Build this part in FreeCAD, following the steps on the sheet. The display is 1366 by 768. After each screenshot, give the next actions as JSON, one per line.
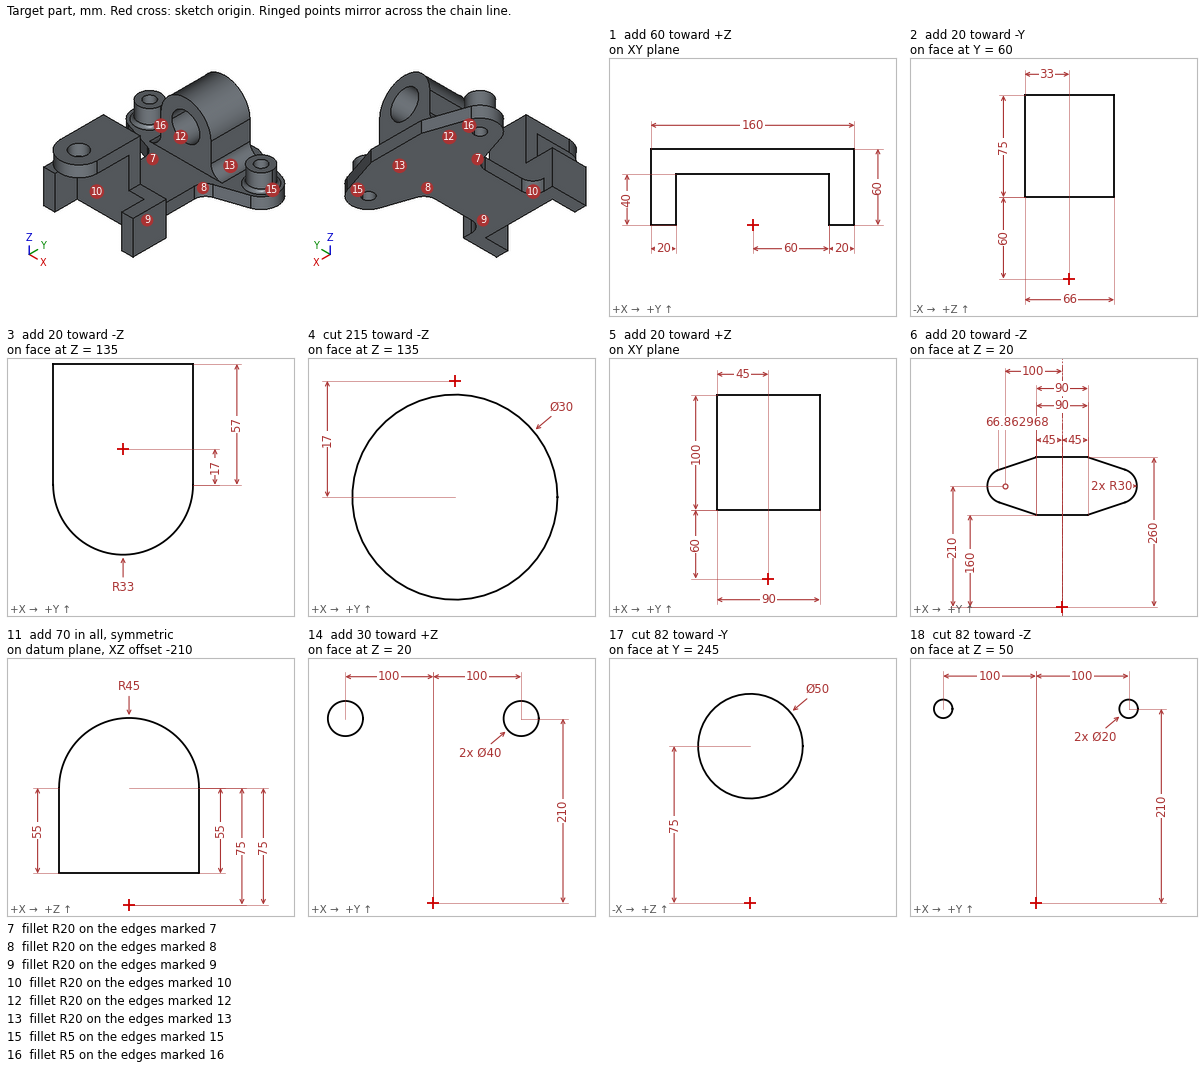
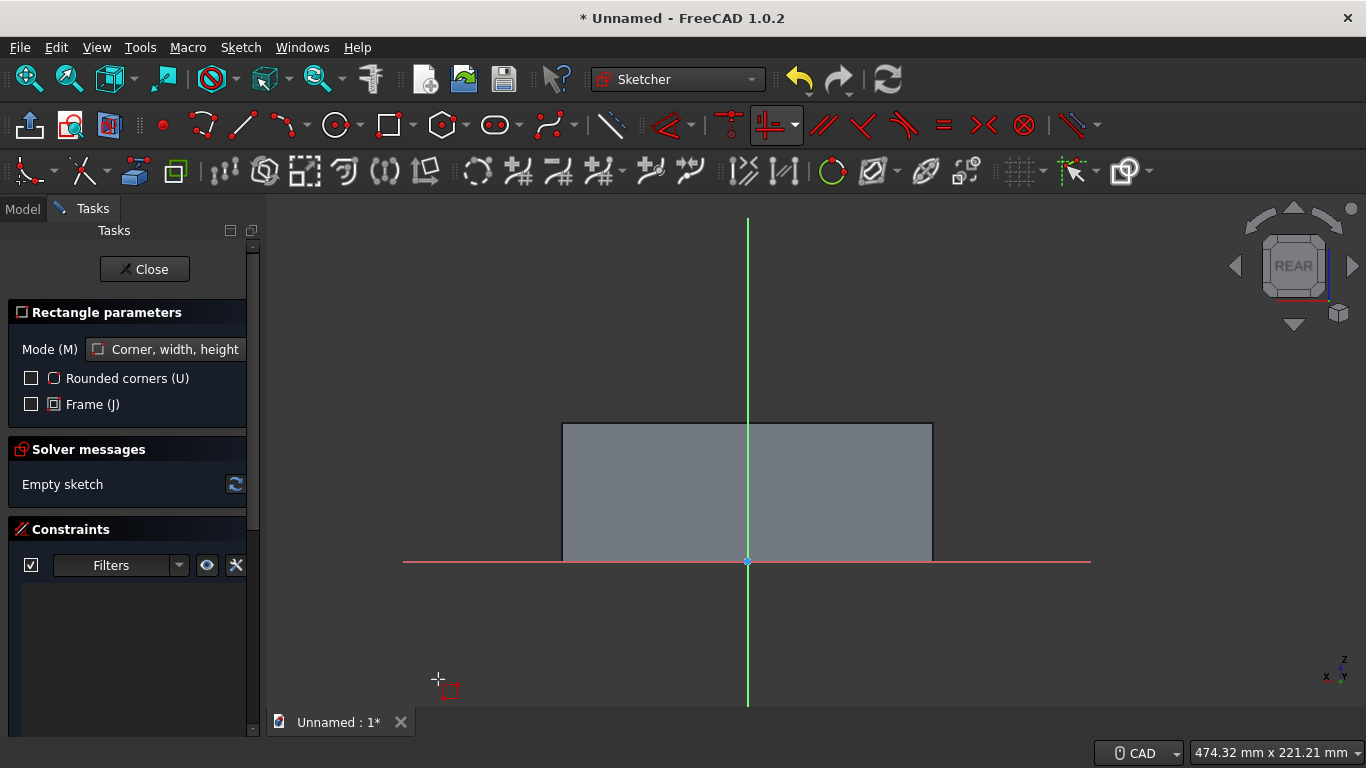
{"action": "left_click", "coordinate": [671, 249]}
{"action": "left_click", "coordinate": [824, 423]}
{"action": "key", "text": "Escape"}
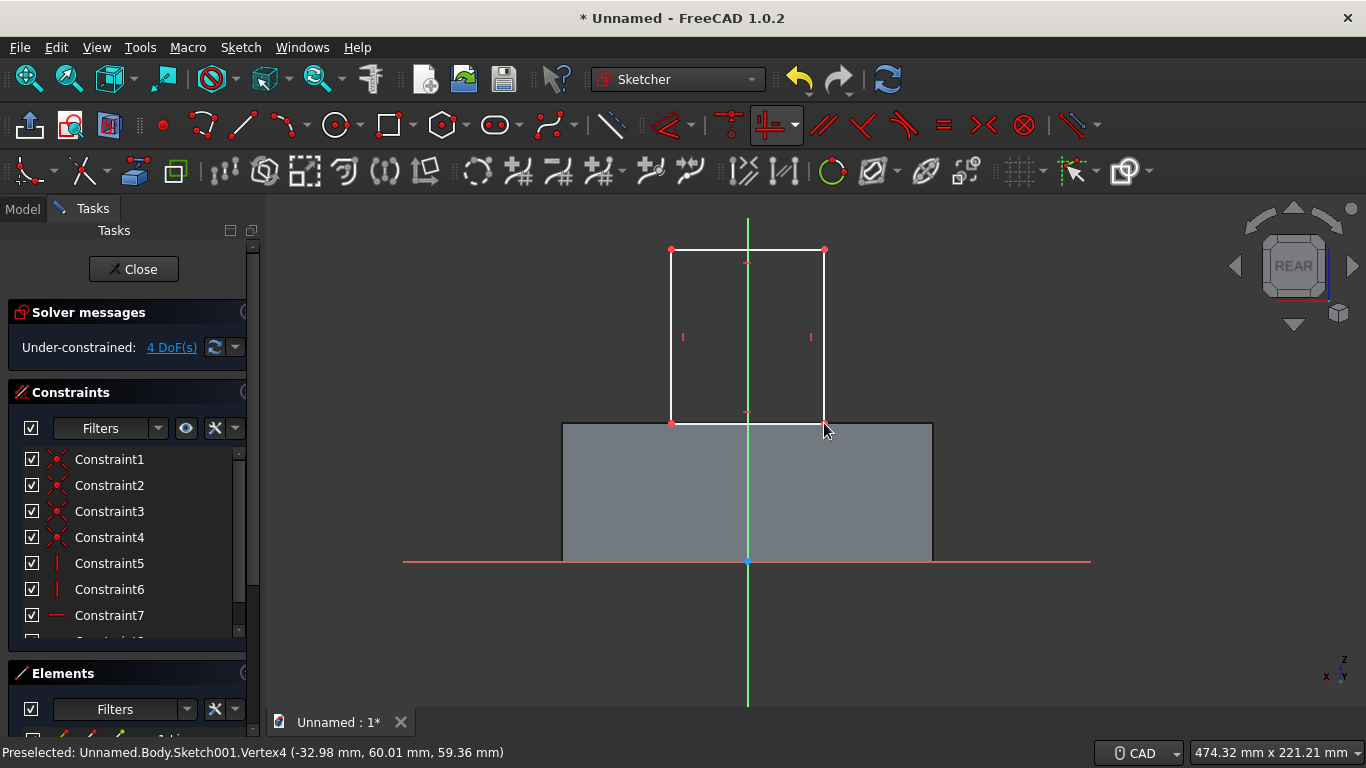
{"action": "left_click", "coordinate": [666, 126]}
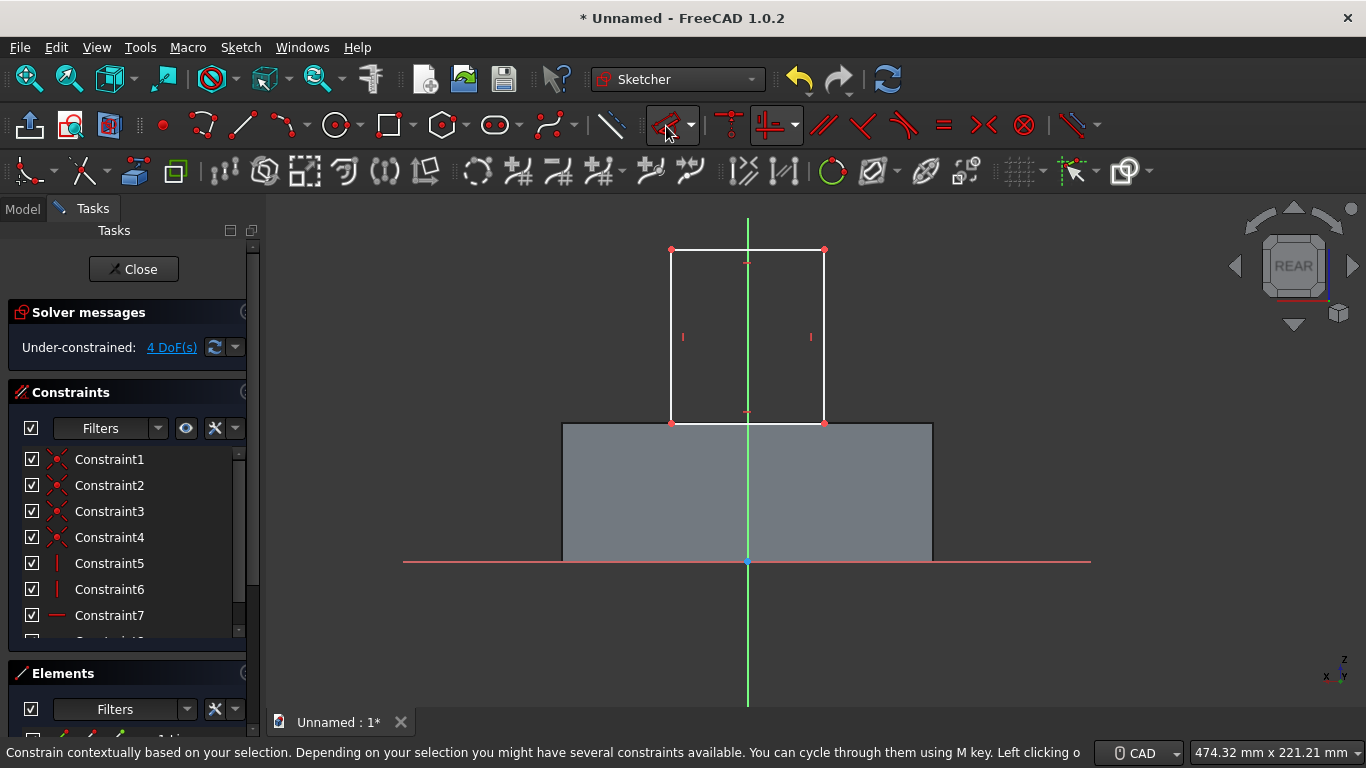
{"action": "left_click", "coordinate": [671, 302]}
{"action": "left_click", "coordinate": [637, 337]}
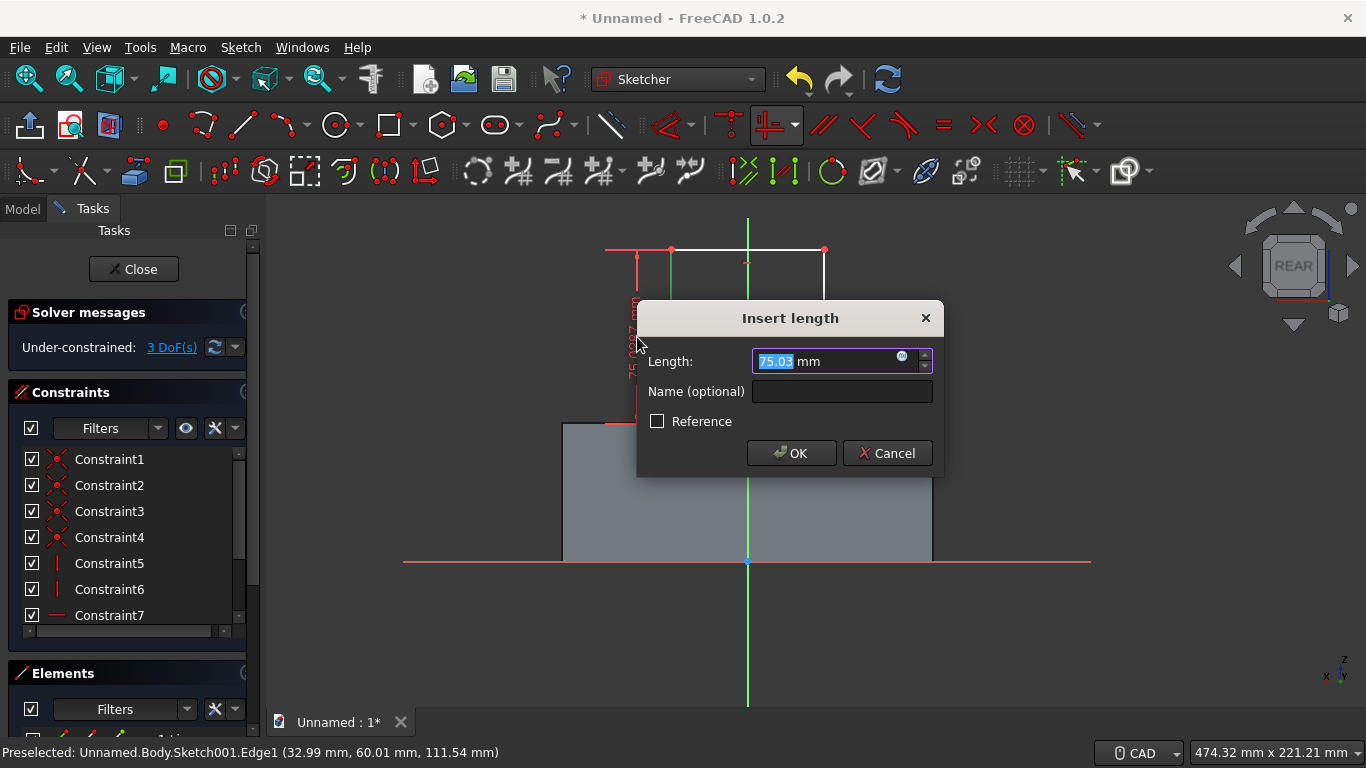
{"action": "type", "text": "75"}
{"action": "key", "text": "Return"}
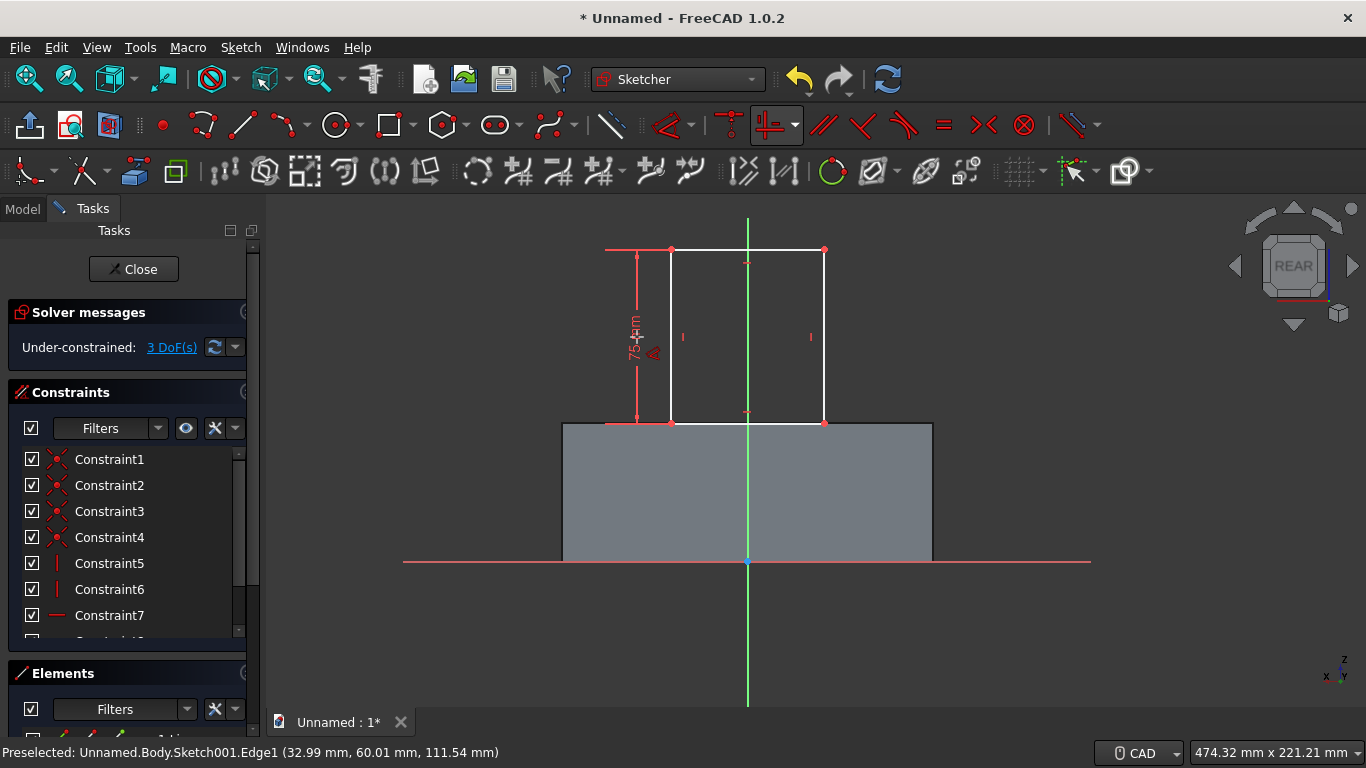
{"action": "left_click", "coordinate": [717, 424]}
{"action": "left_click", "coordinate": [712, 458]}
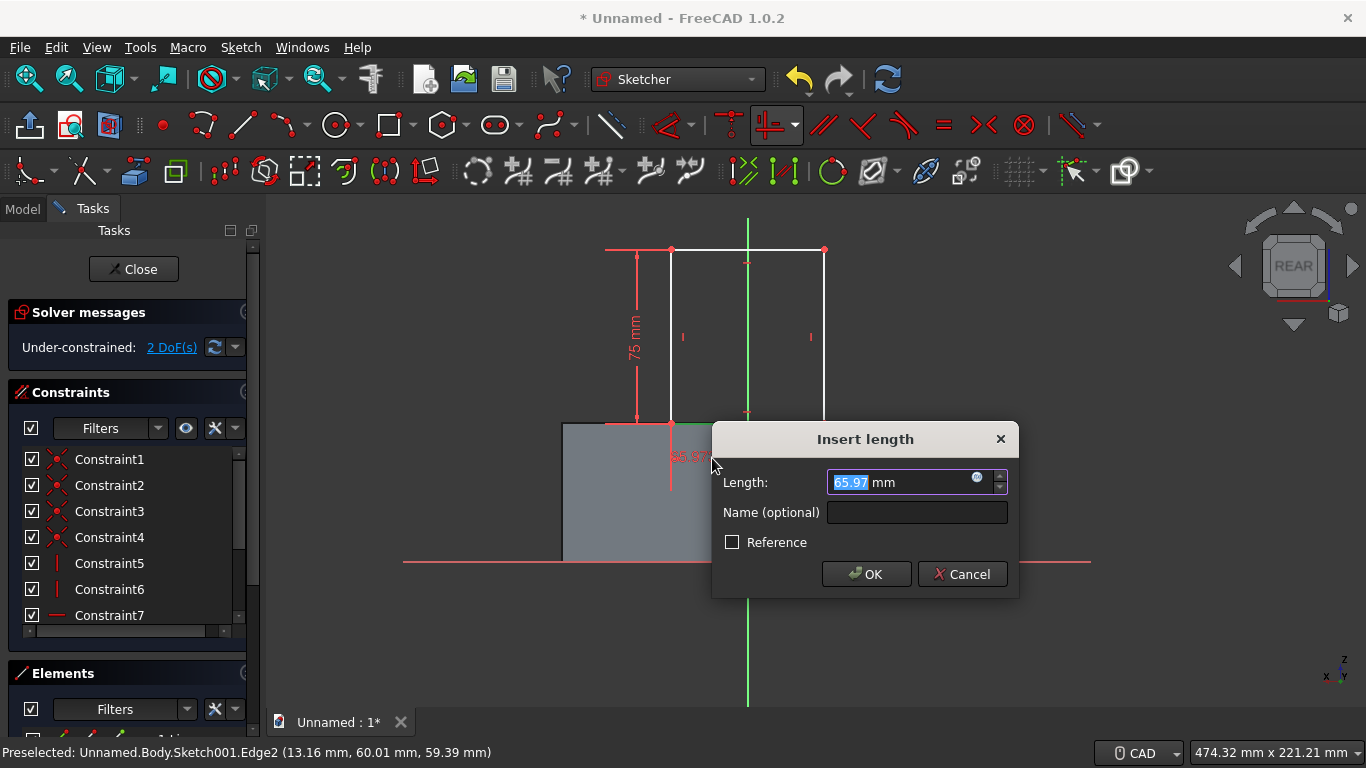
{"action": "type", "text": "66"}
{"action": "key", "text": "Return"}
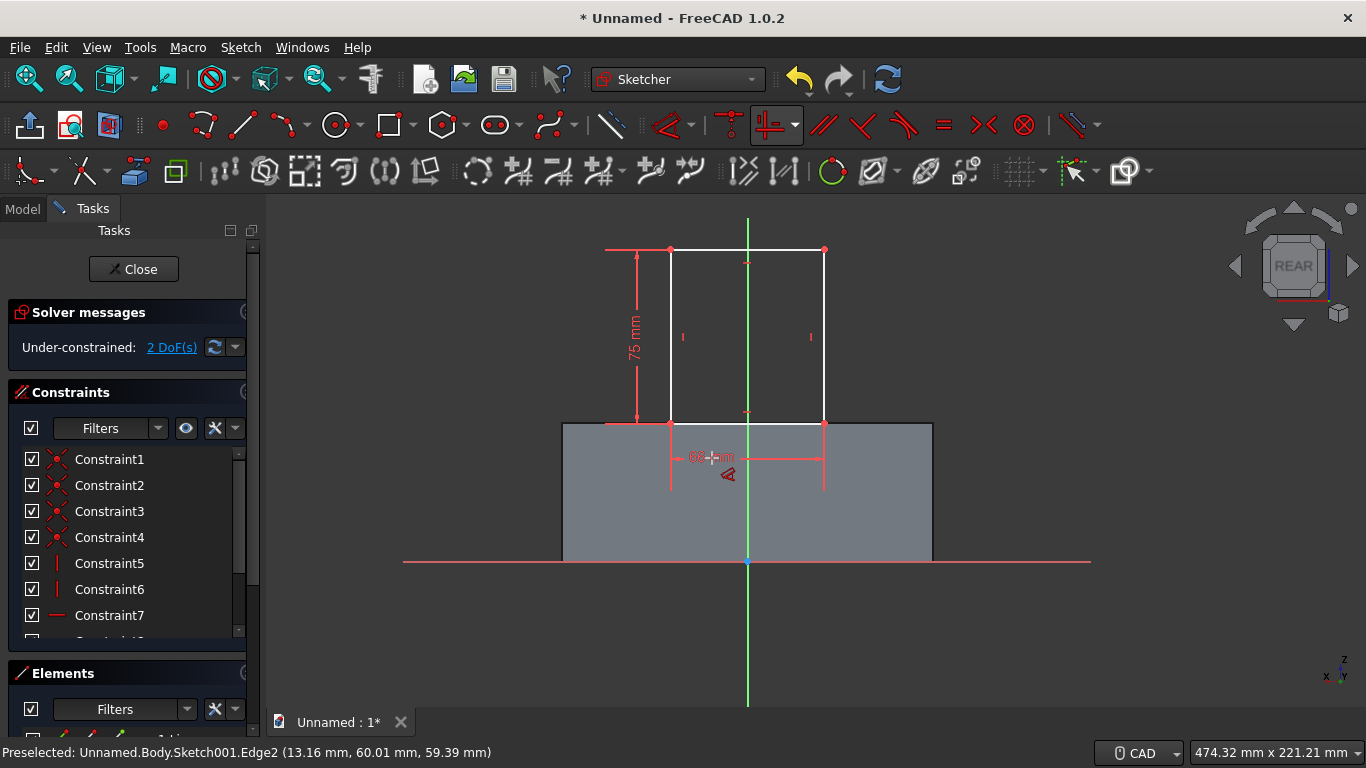
{"action": "left_click", "coordinate": [671, 250]}
{"action": "left_click", "coordinate": [709, 596]}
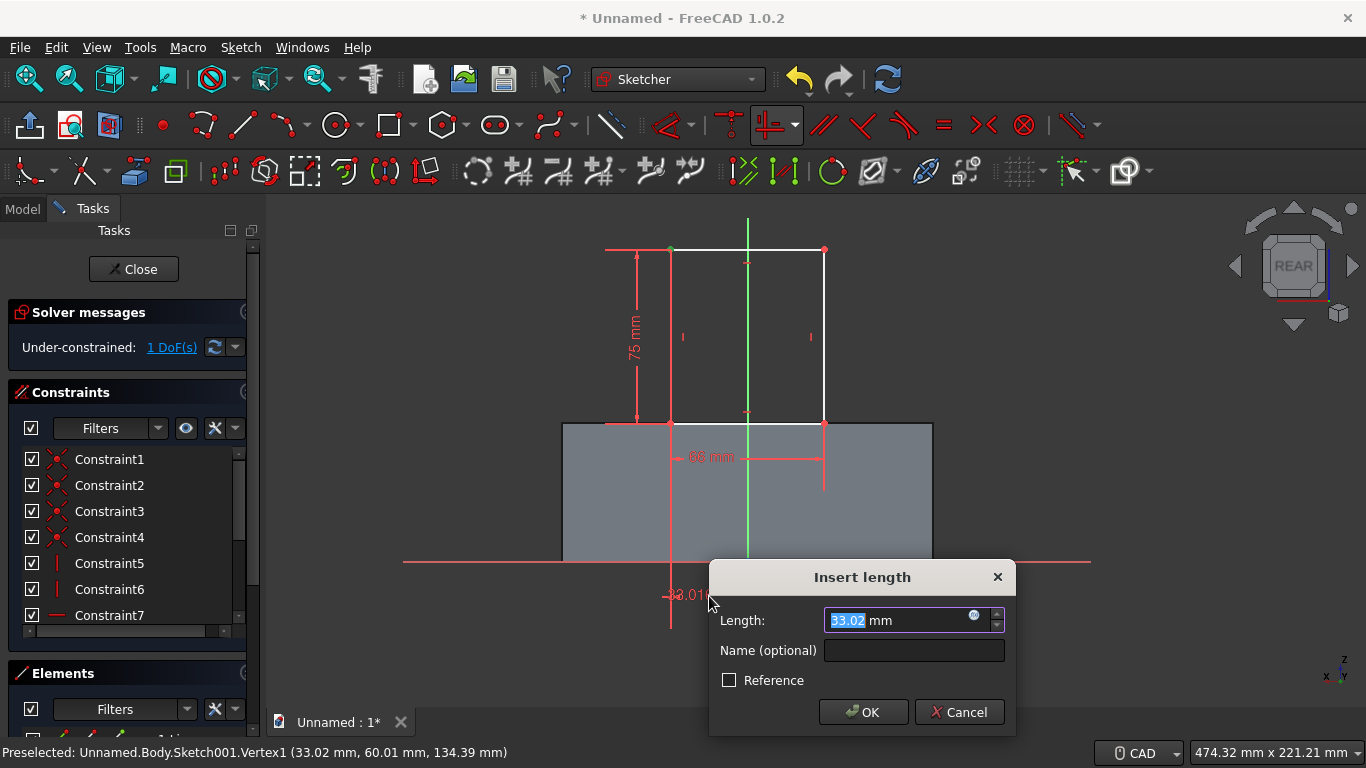
{"action": "type", "text": "33"}
{"action": "key", "text": "Return"}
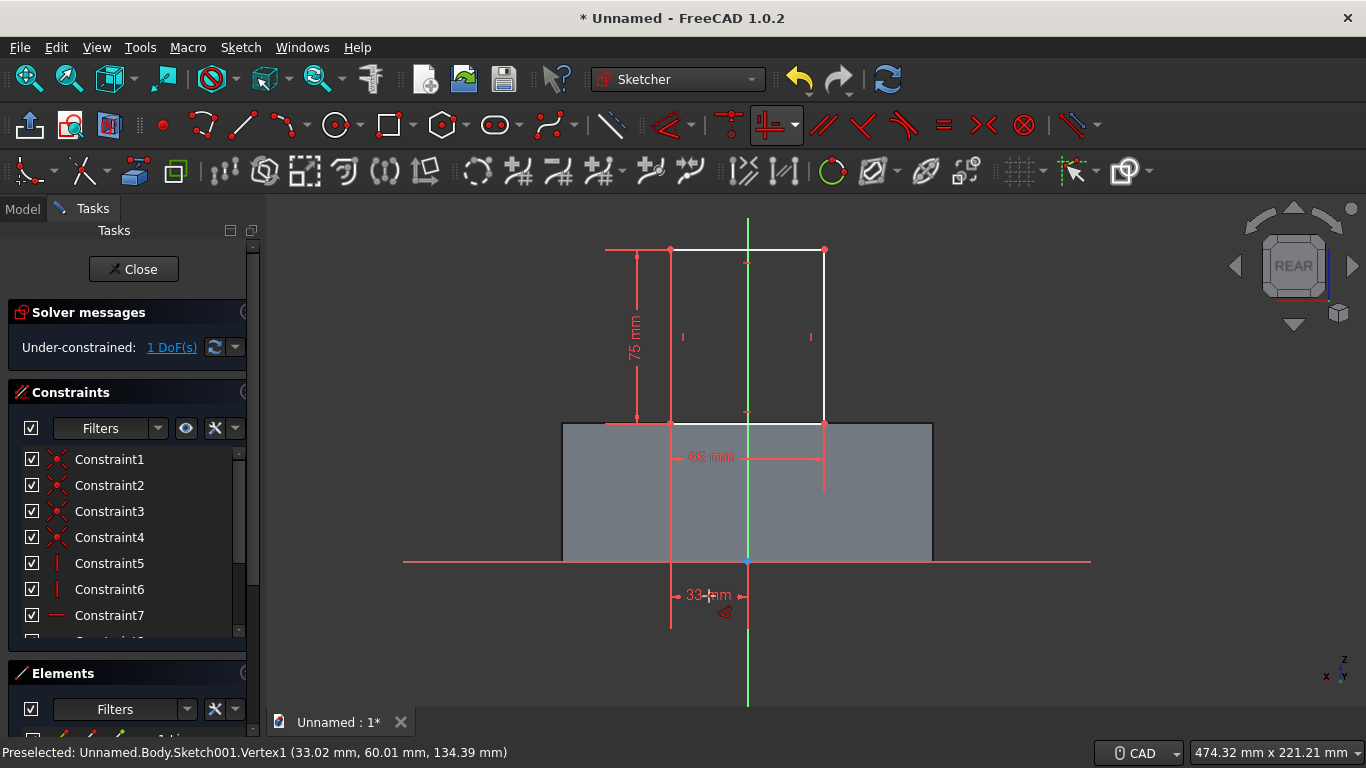
{"action": "left_click", "coordinate": [671, 424]}
{"action": "left_click", "coordinate": [637, 493]}